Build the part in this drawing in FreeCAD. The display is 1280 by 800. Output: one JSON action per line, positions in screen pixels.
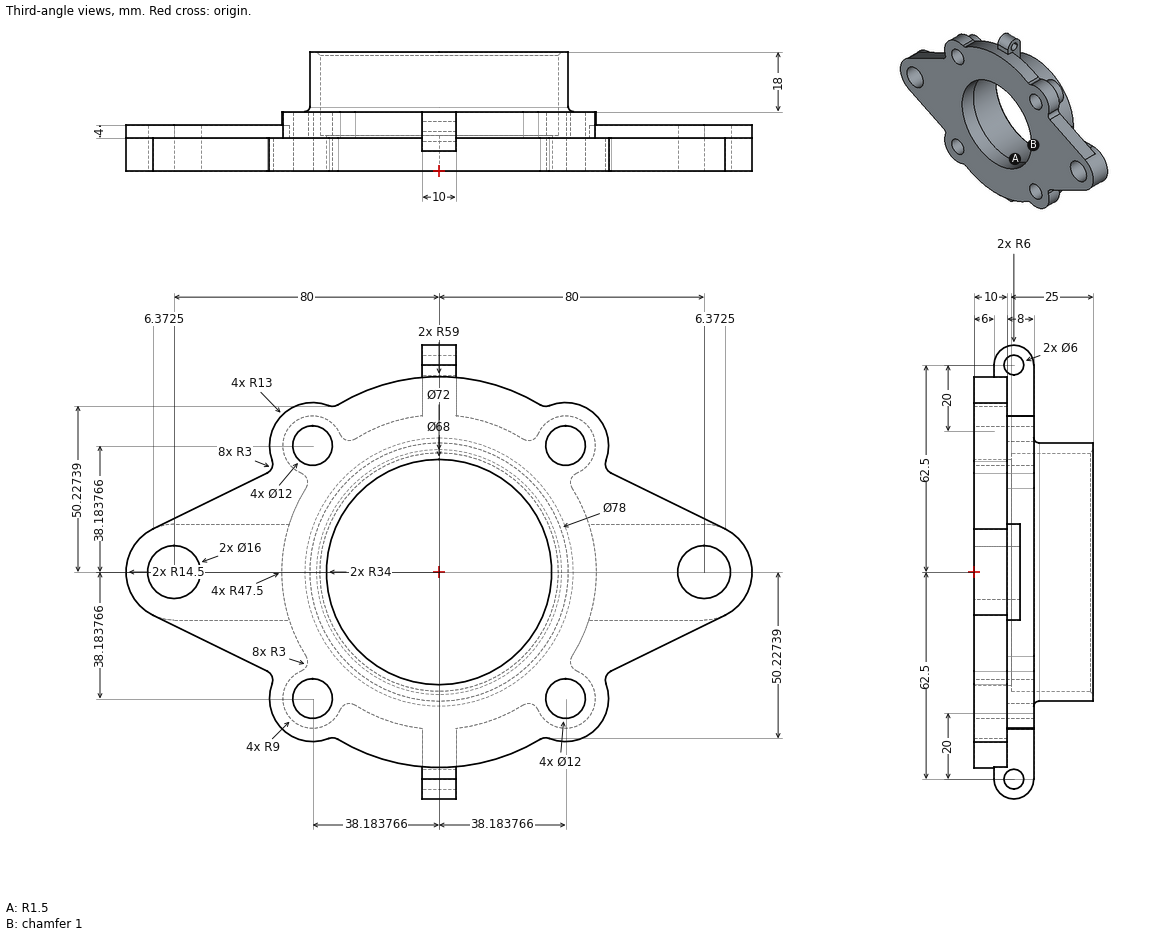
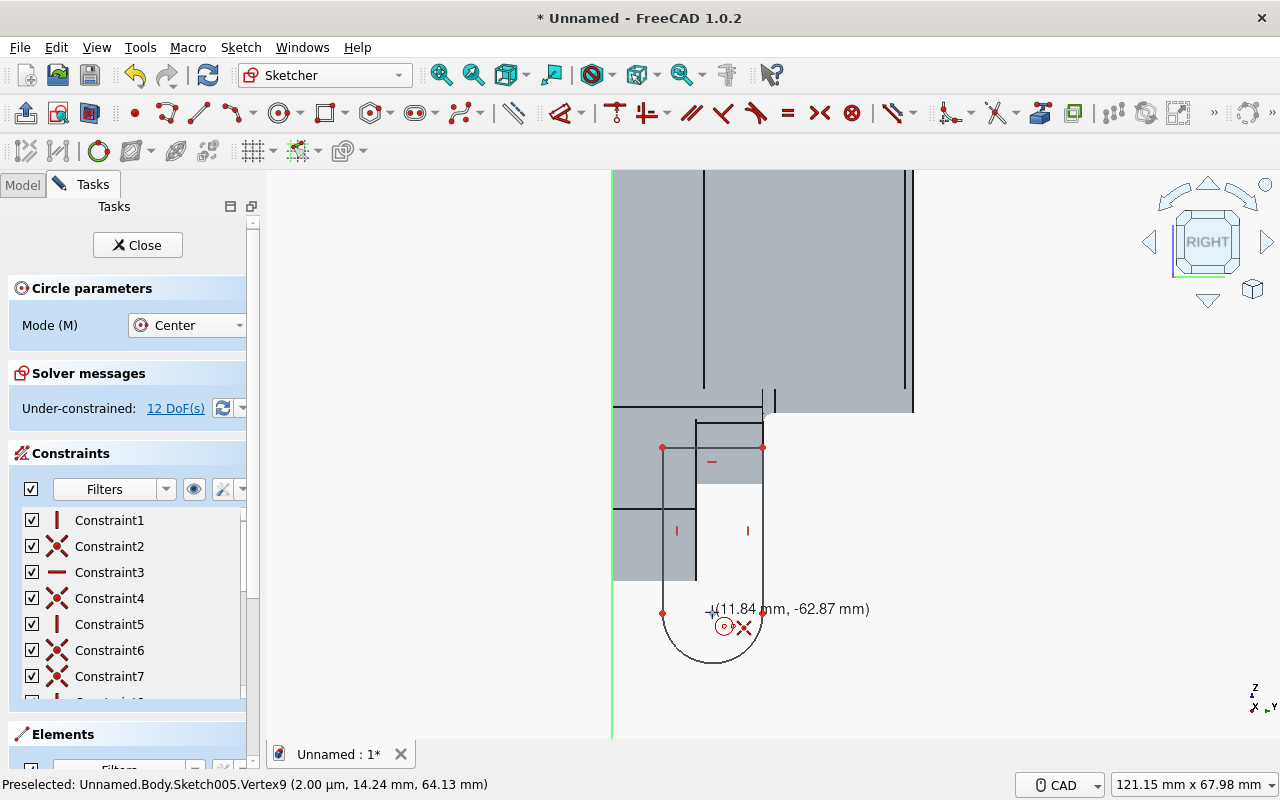
{"action": "left_click", "coordinate": [712, 610]}
{"action": "mouse_move", "coordinate": [730, 593]}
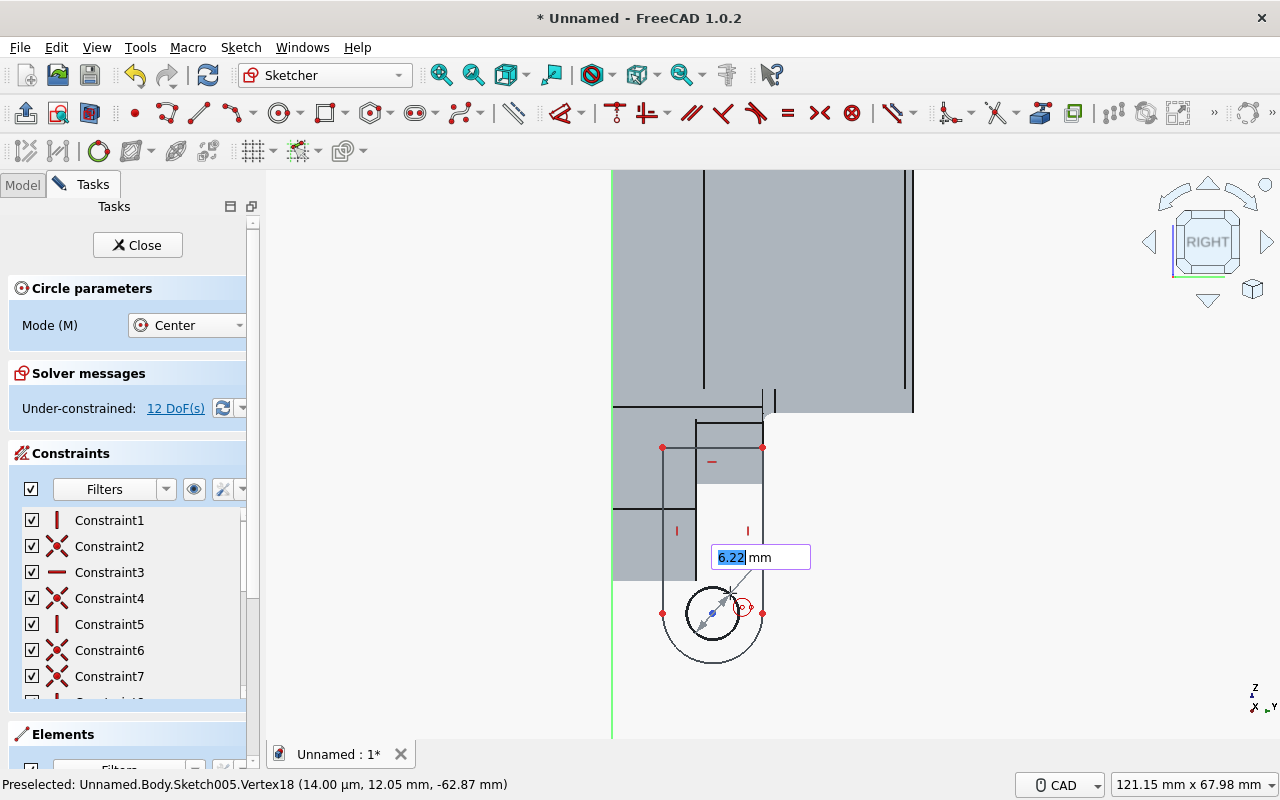
{"action": "type", "text": "6"}
{"action": "key", "text": "Return"}
{"action": "key", "text": "Escape"}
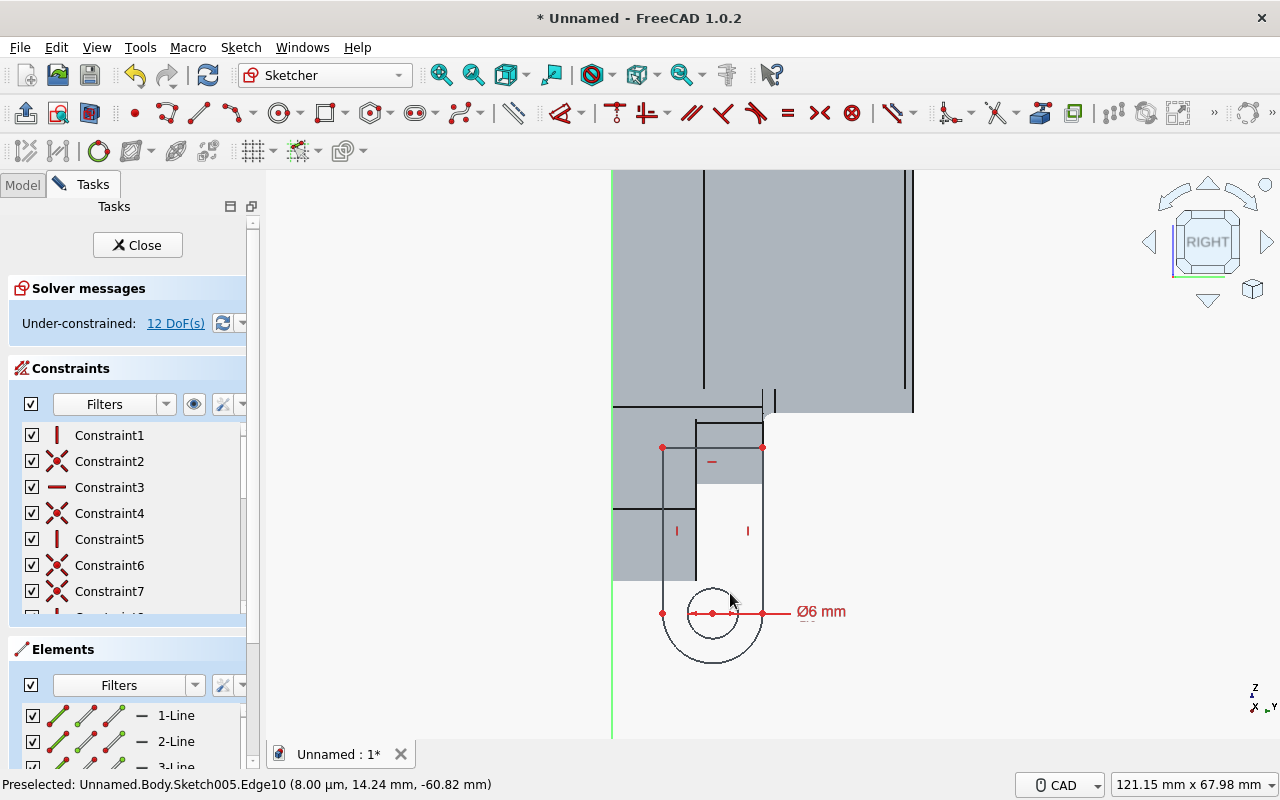
{"action": "scroll", "coordinate": [712, 613], "scroll_direction": "down", "scroll_amount": 6}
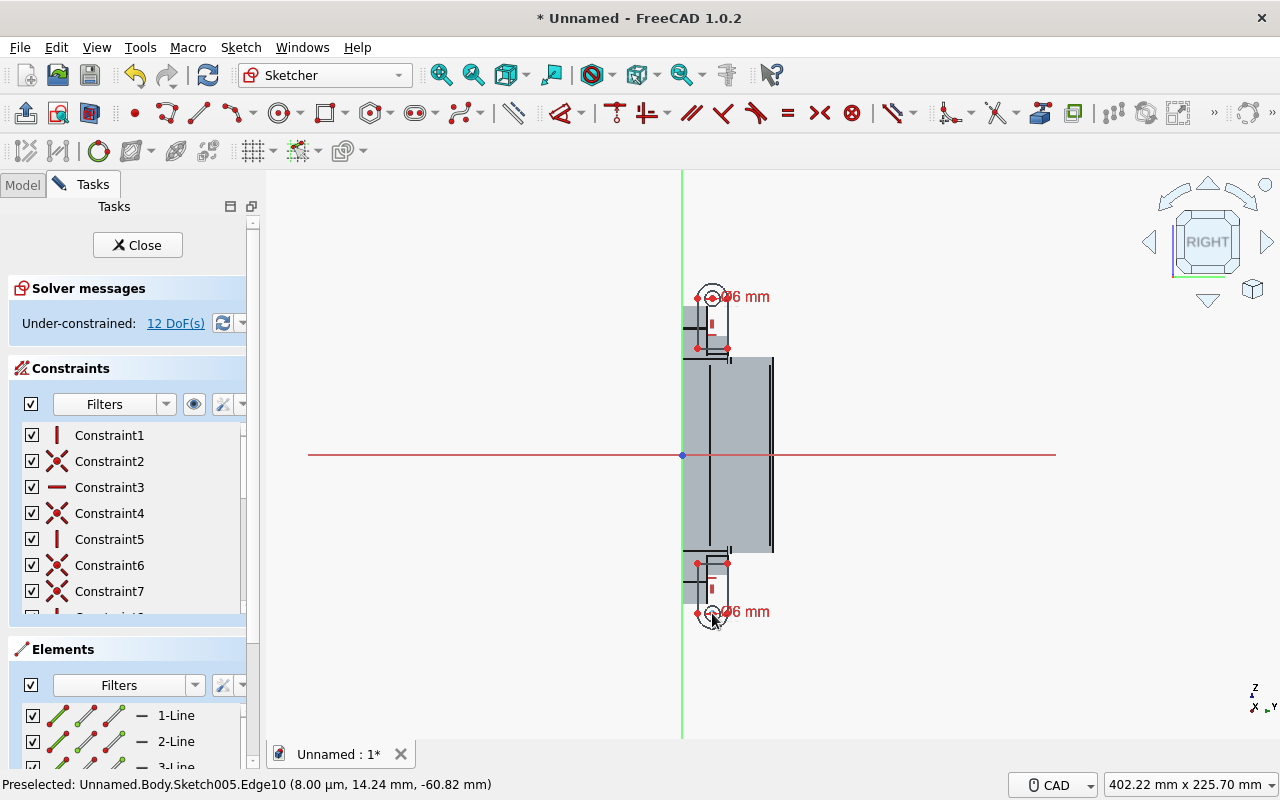
{"action": "left_click", "coordinate": [698, 314]}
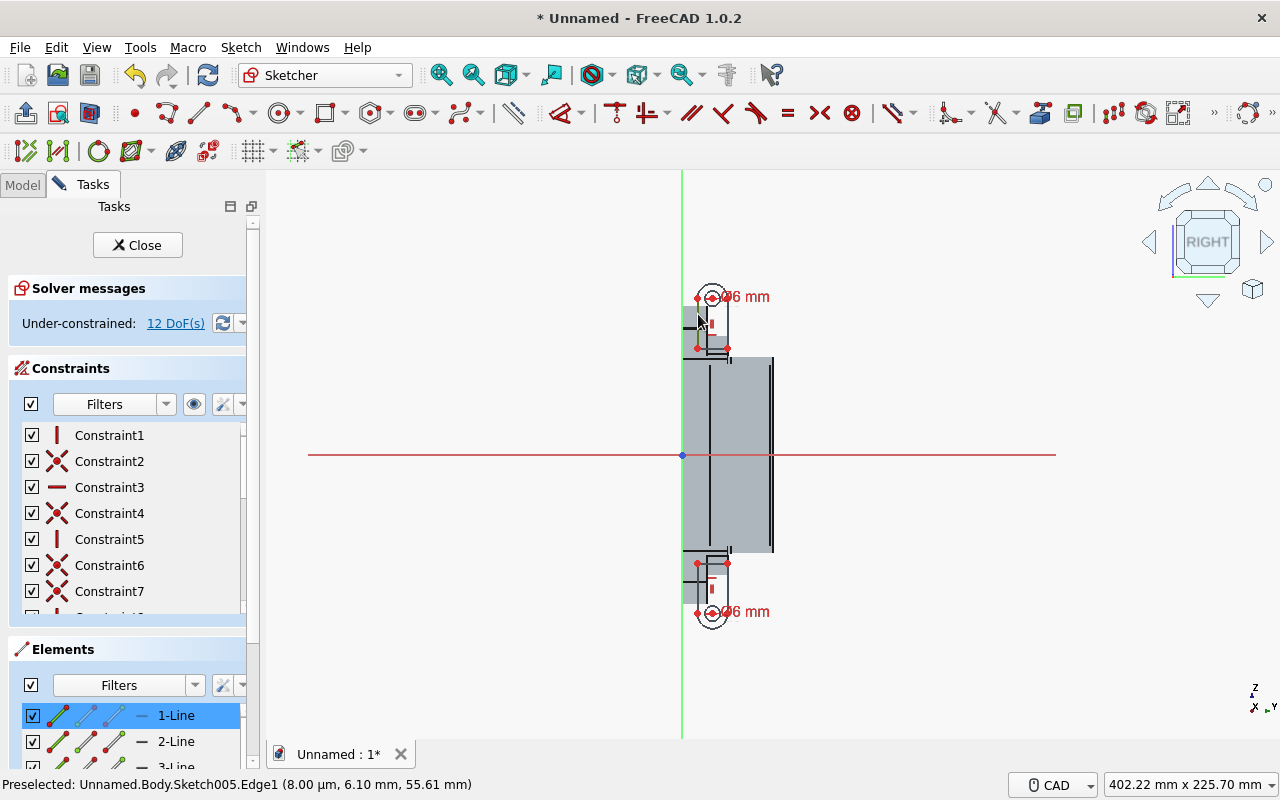
{"action": "scroll", "coordinate": [704, 287], "scroll_direction": "up", "scroll_amount": 4}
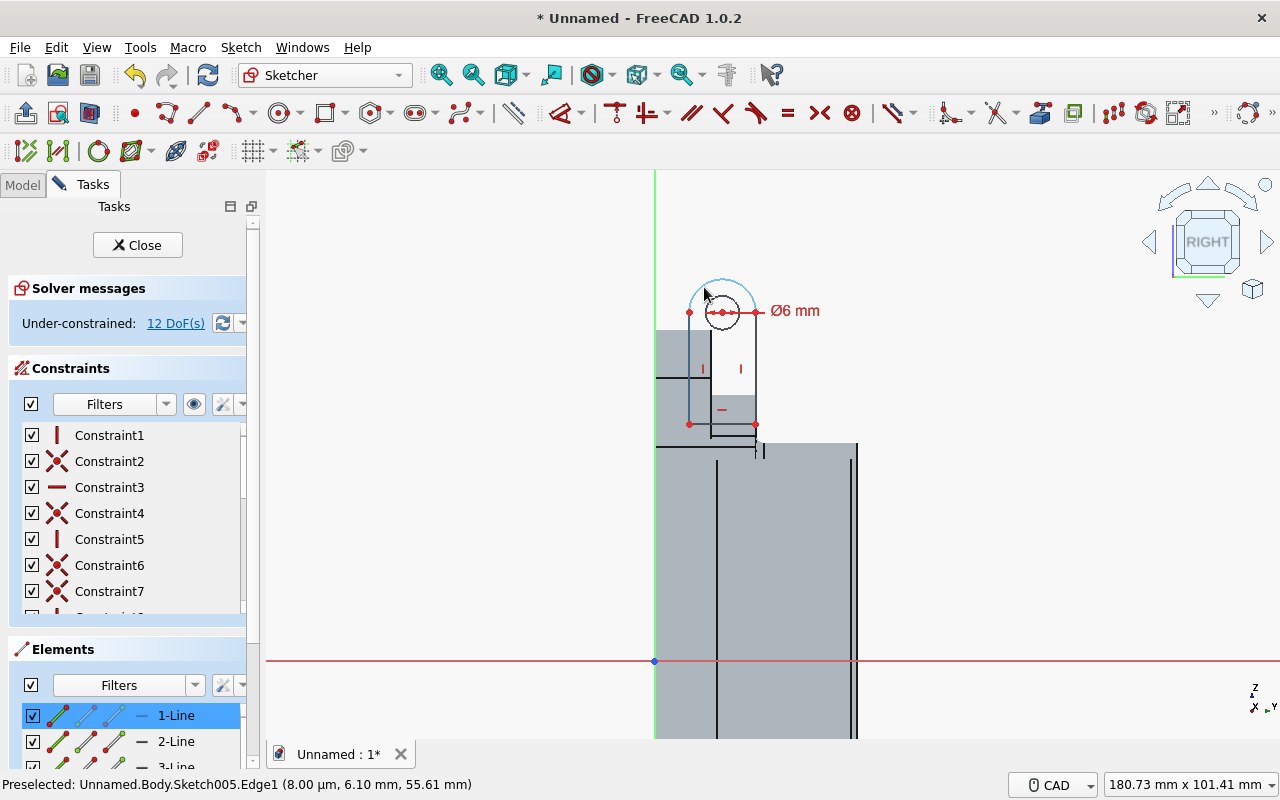
{"action": "left_click", "coordinate": [703, 286]}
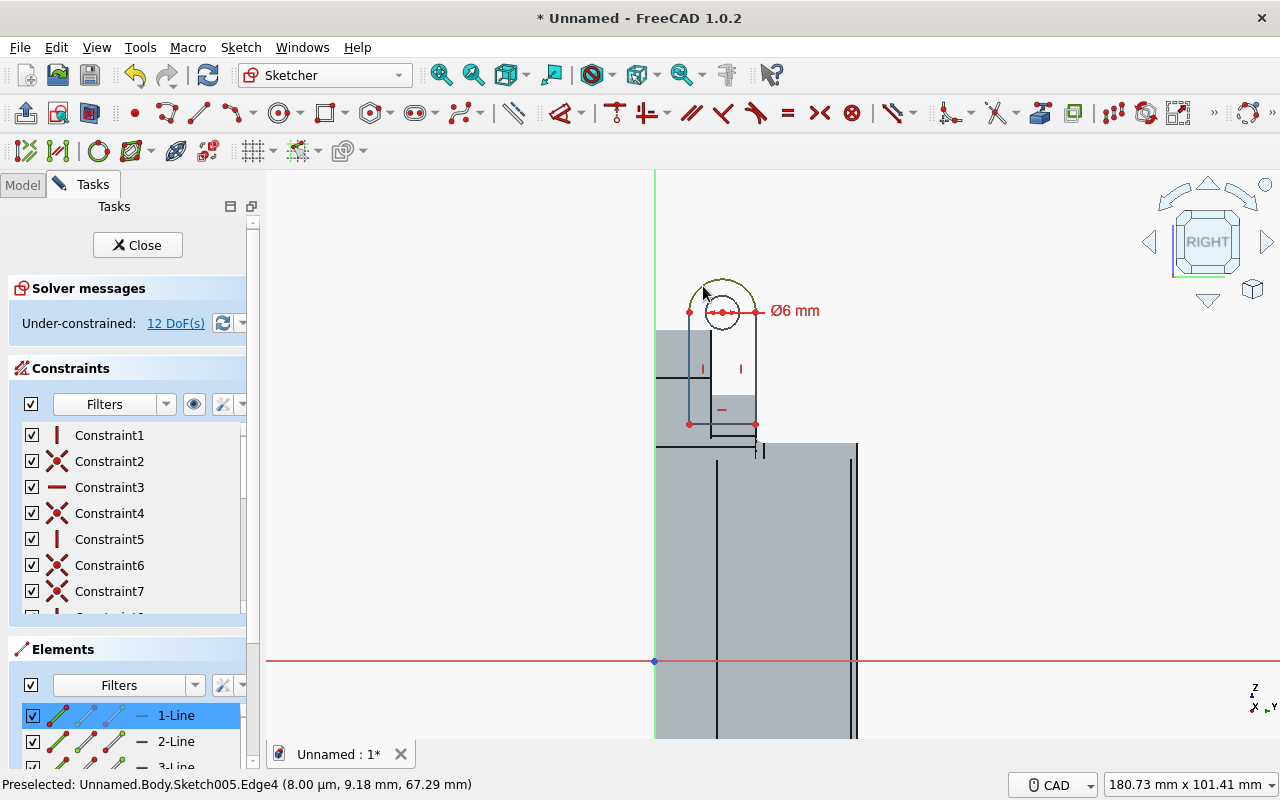
{"action": "left_click", "coordinate": [756, 114]}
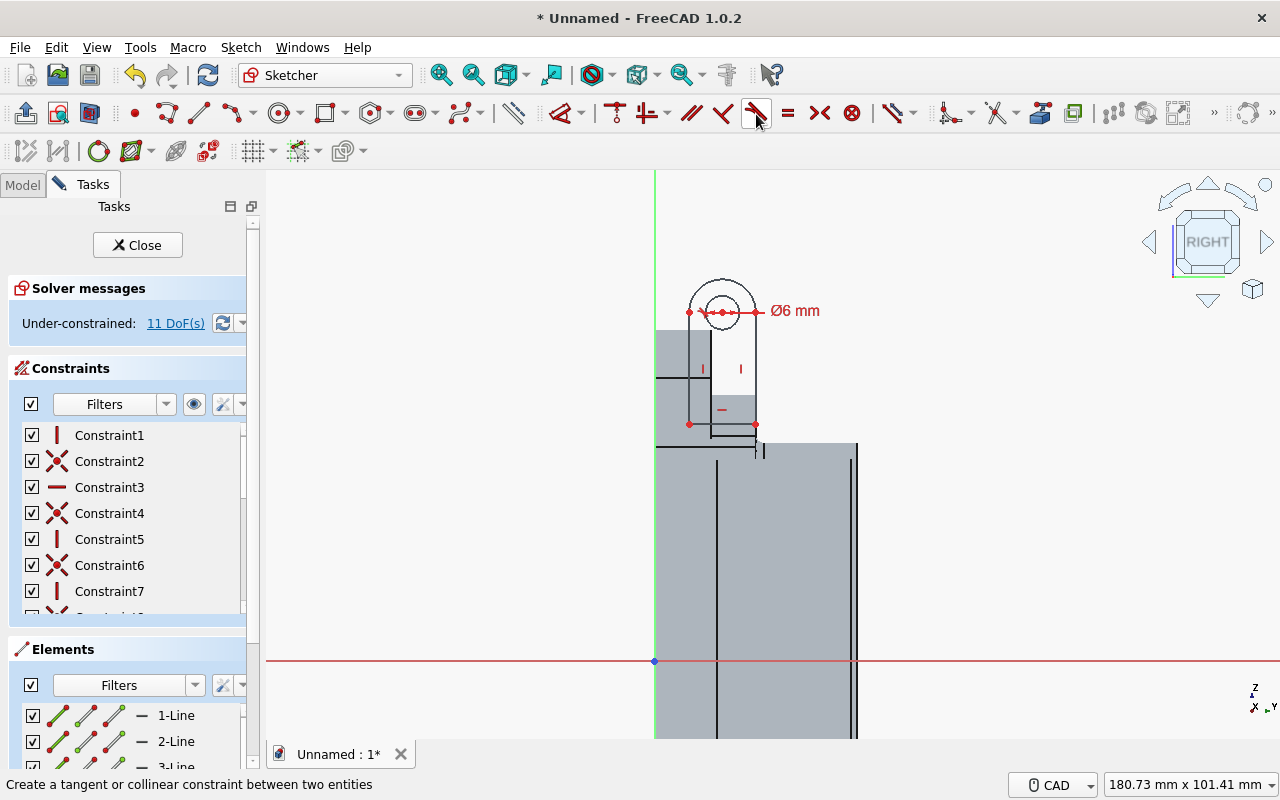
{"action": "left_click", "coordinate": [756, 391]}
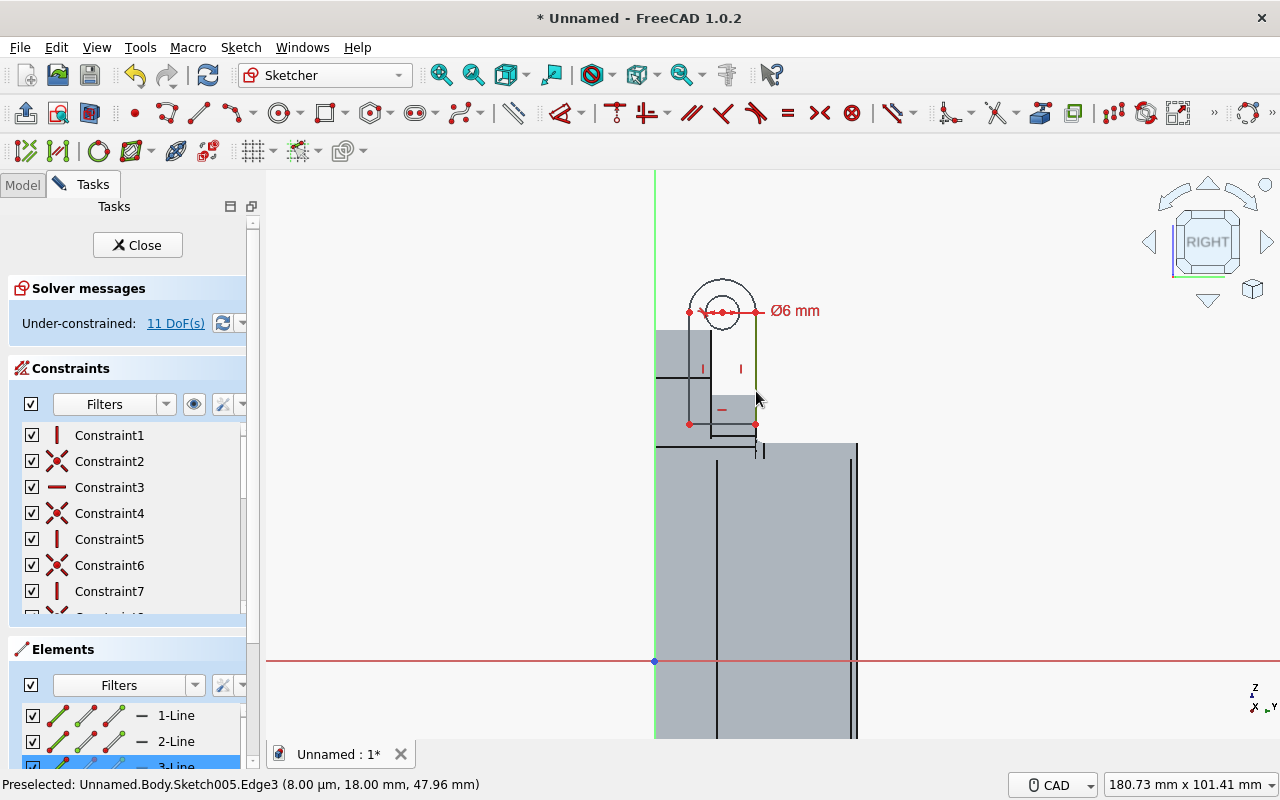
{"action": "left_click", "coordinate": [742, 286]}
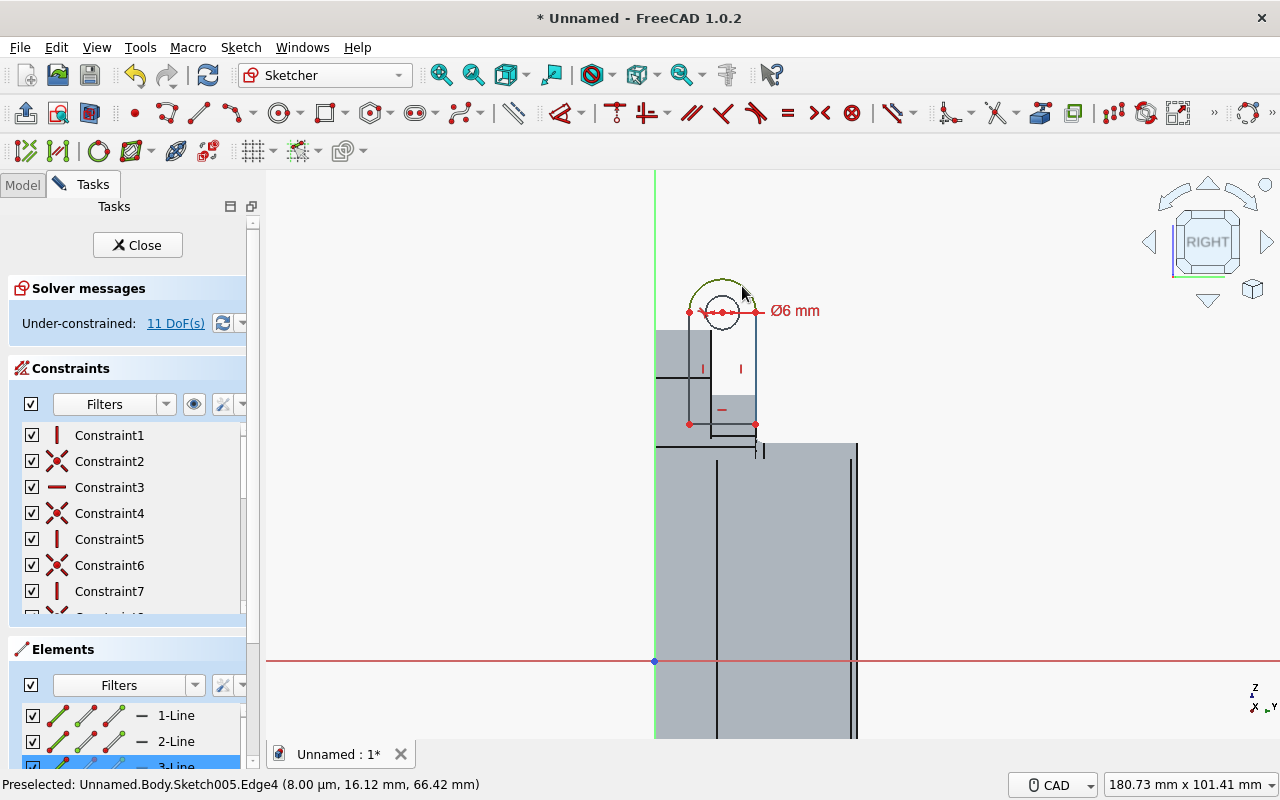
{"action": "left_click", "coordinate": [756, 114]}